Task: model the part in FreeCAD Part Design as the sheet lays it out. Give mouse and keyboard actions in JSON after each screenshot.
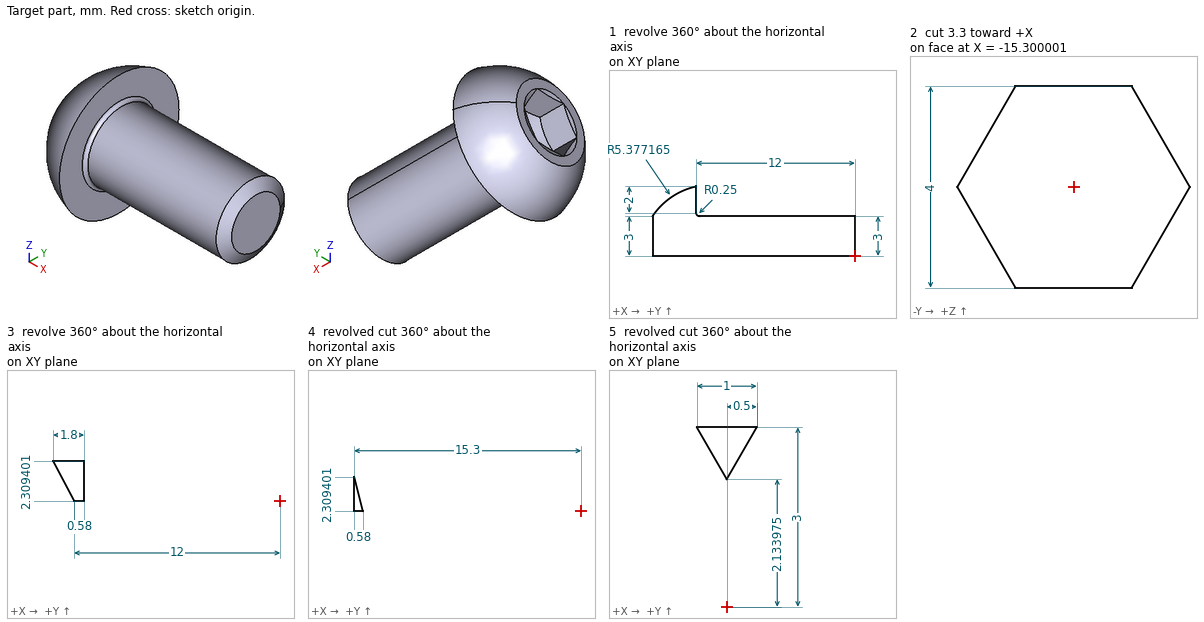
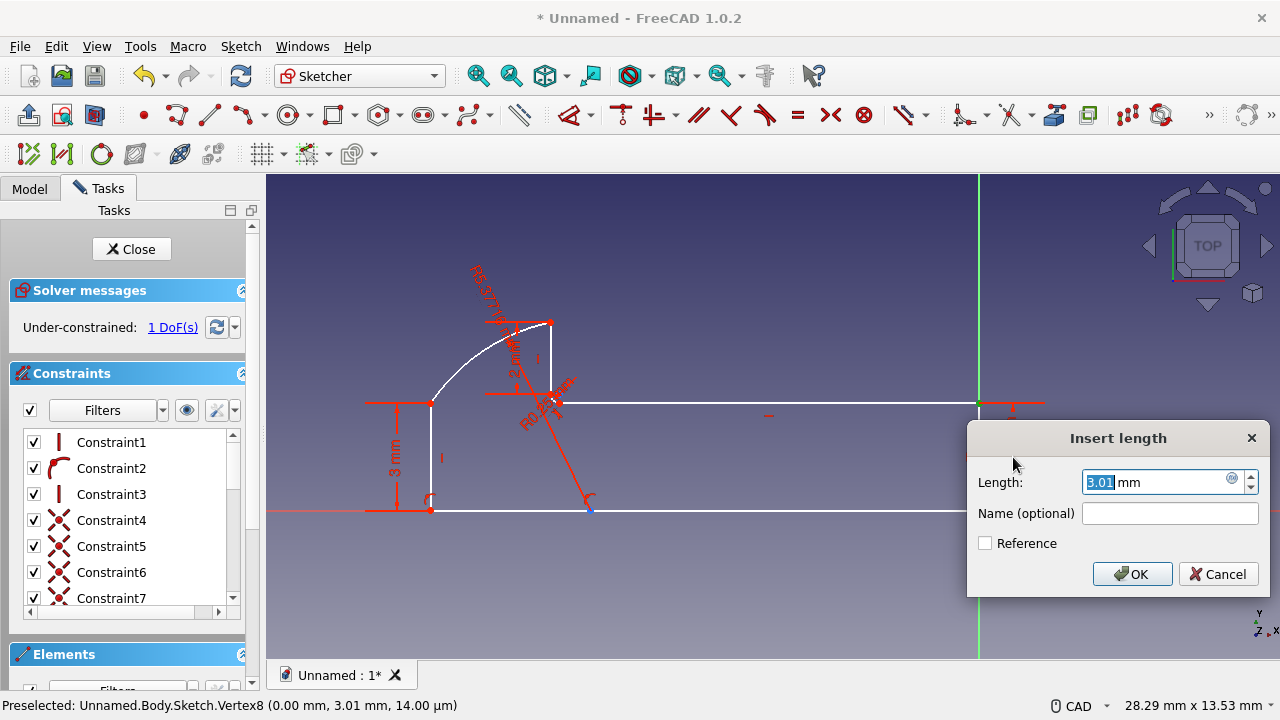
{"action": "type", "text": "3"}
{"action": "key", "text": "Return"}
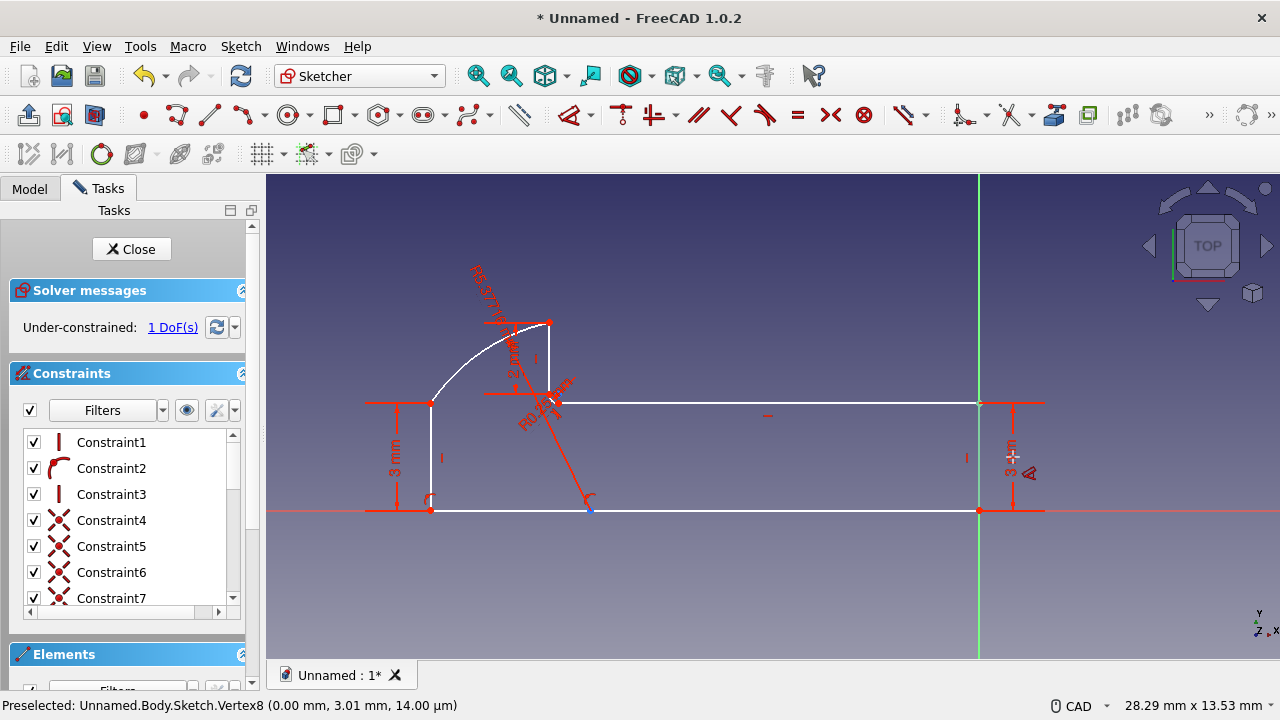
{"action": "scroll", "coordinate": [549, 394], "scroll_direction": "up", "scroll_amount": 2}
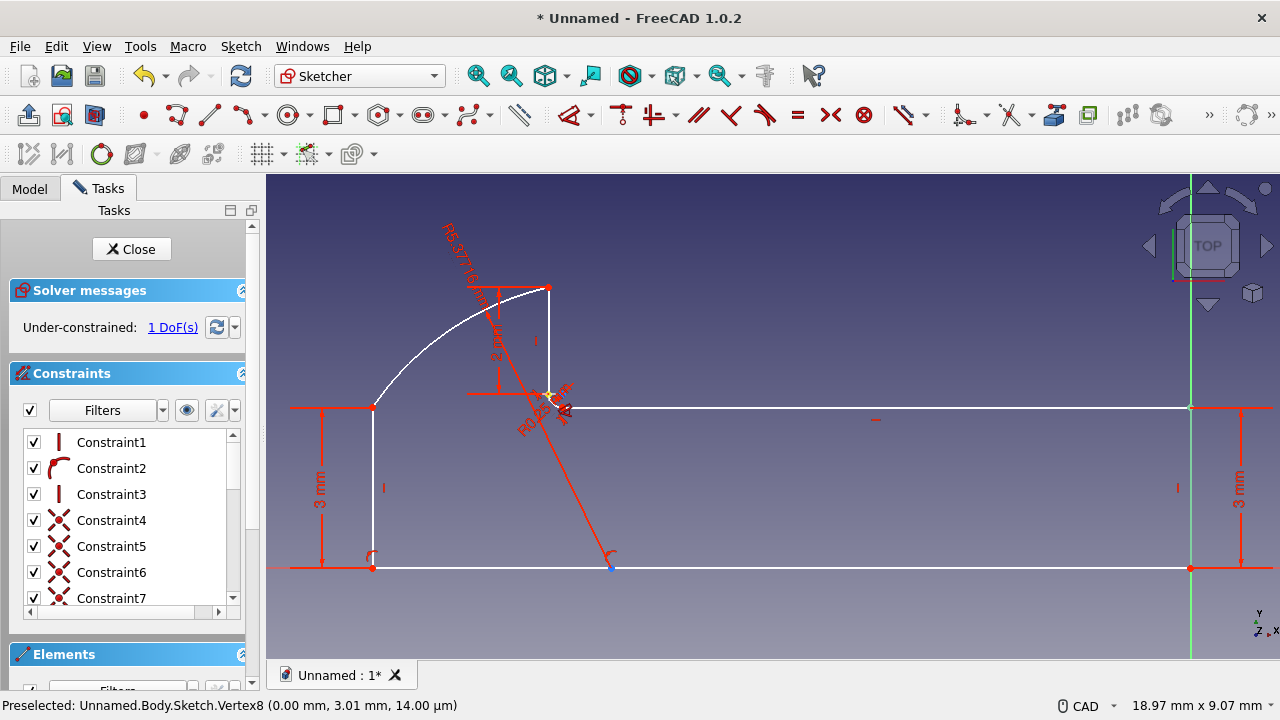
{"action": "left_click", "coordinate": [549, 394]}
{"action": "left_click", "coordinate": [832, 602]}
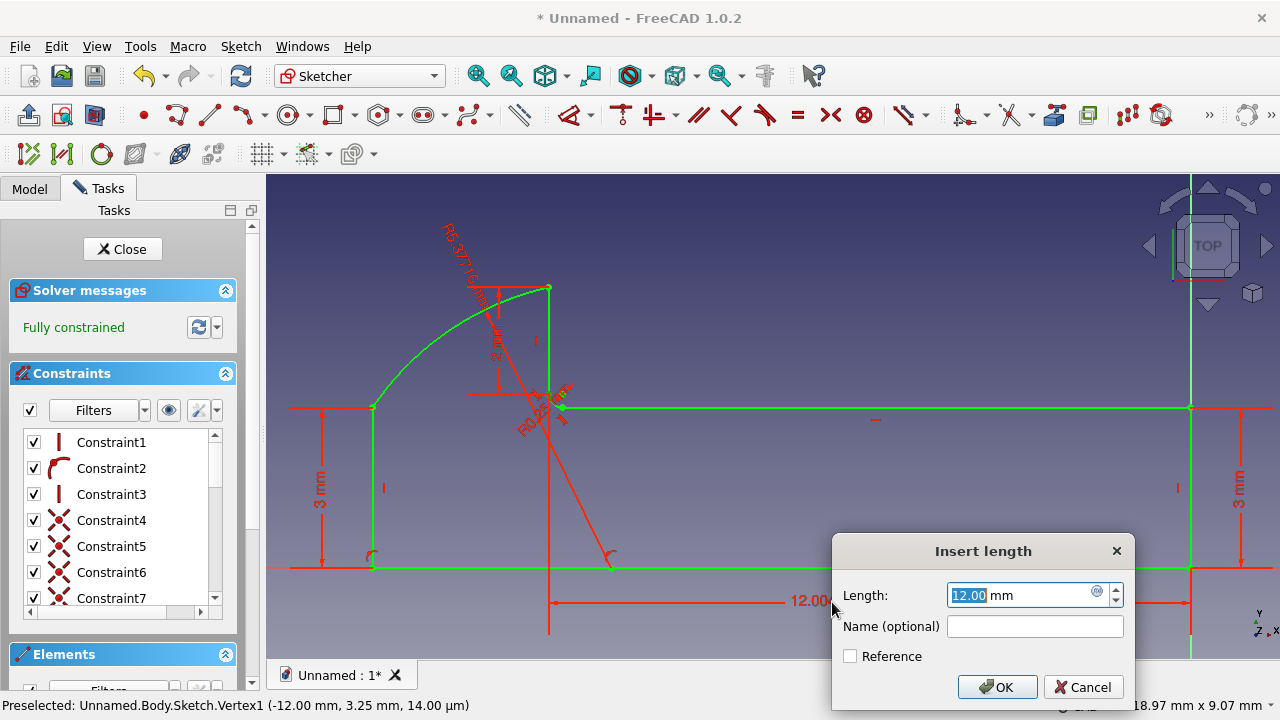
{"action": "type", "text": "12"}
{"action": "key", "text": "Return"}
{"action": "key", "text": "Escape"}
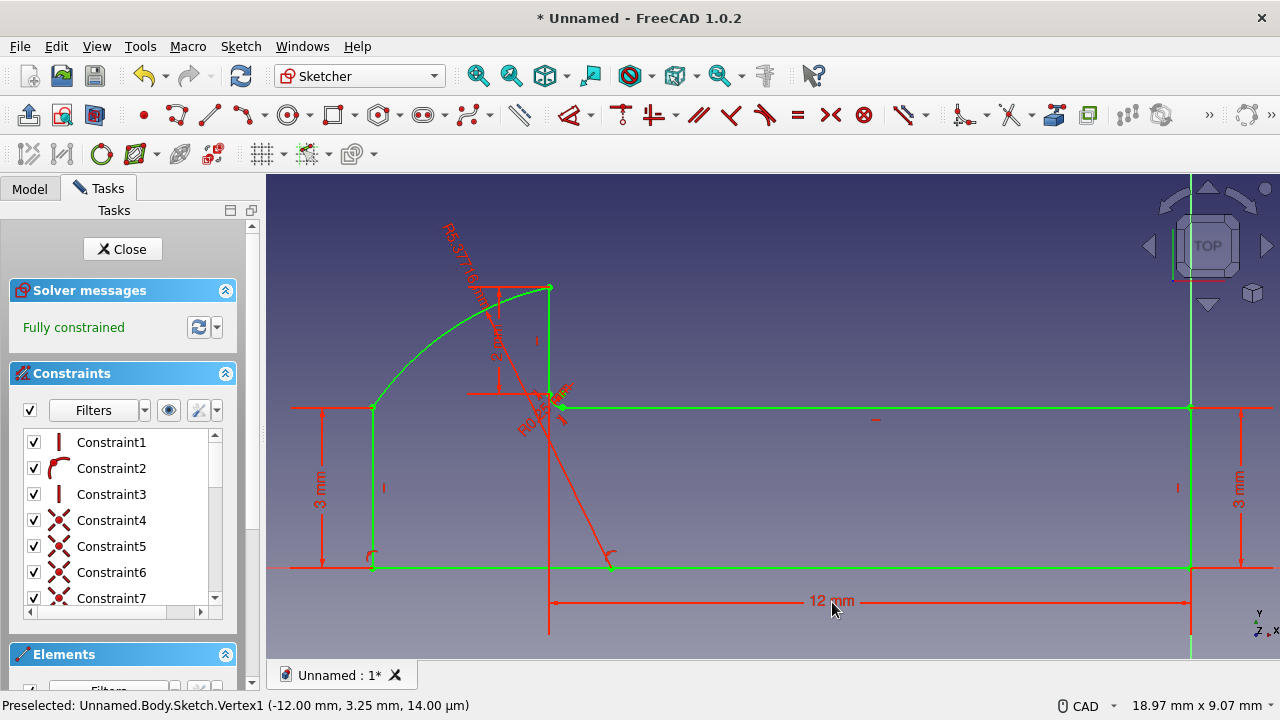
{"action": "left_click", "coordinate": [123, 249]}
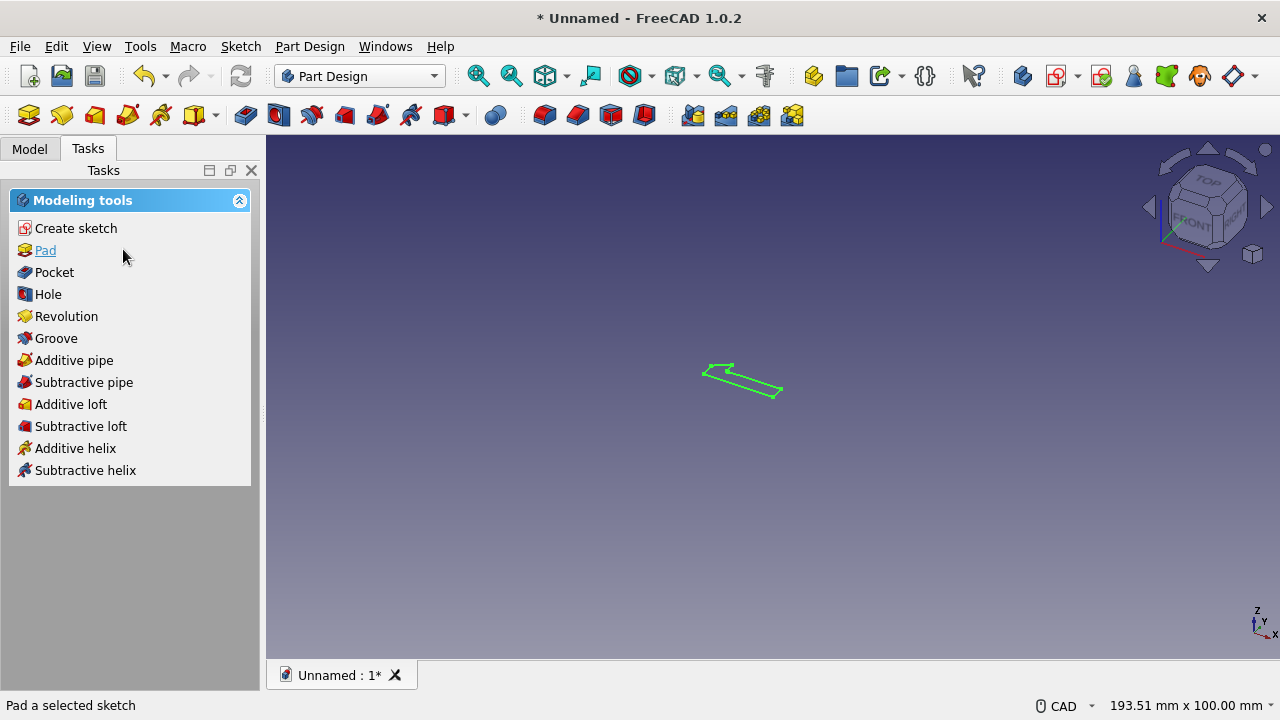
{"action": "left_click", "coordinate": [62, 116]}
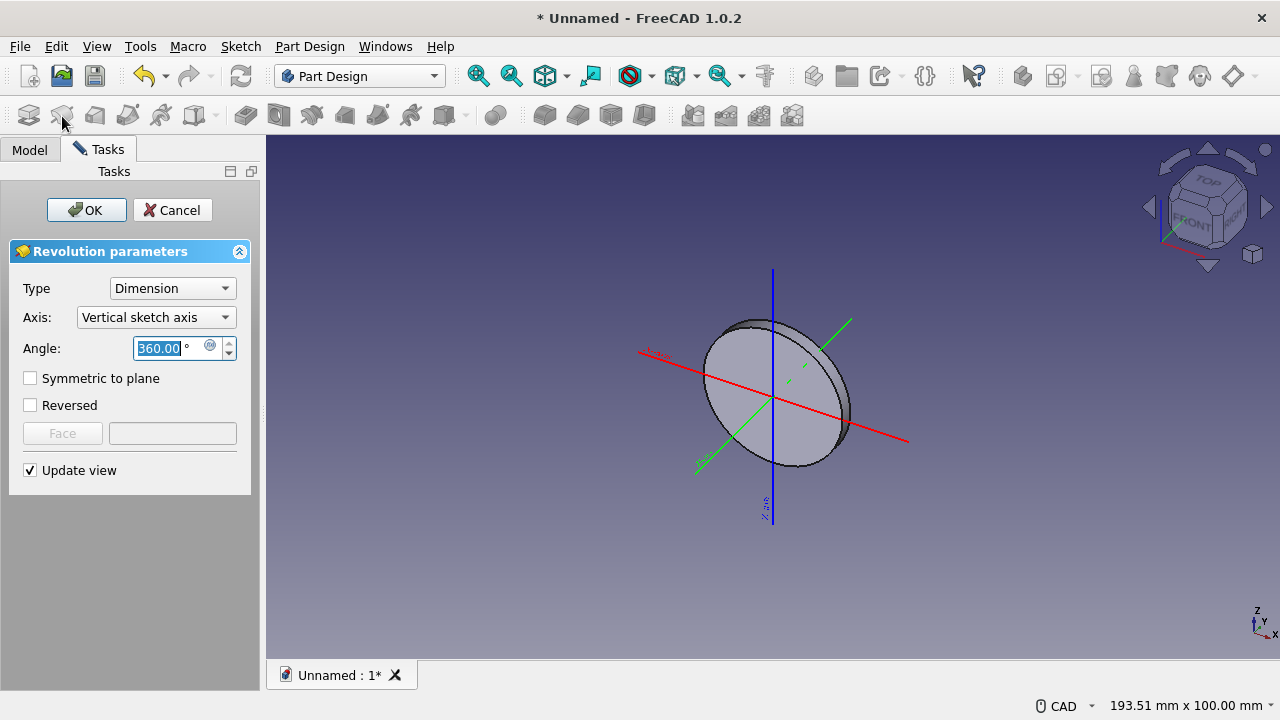
{"action": "left_click", "coordinate": [157, 318]}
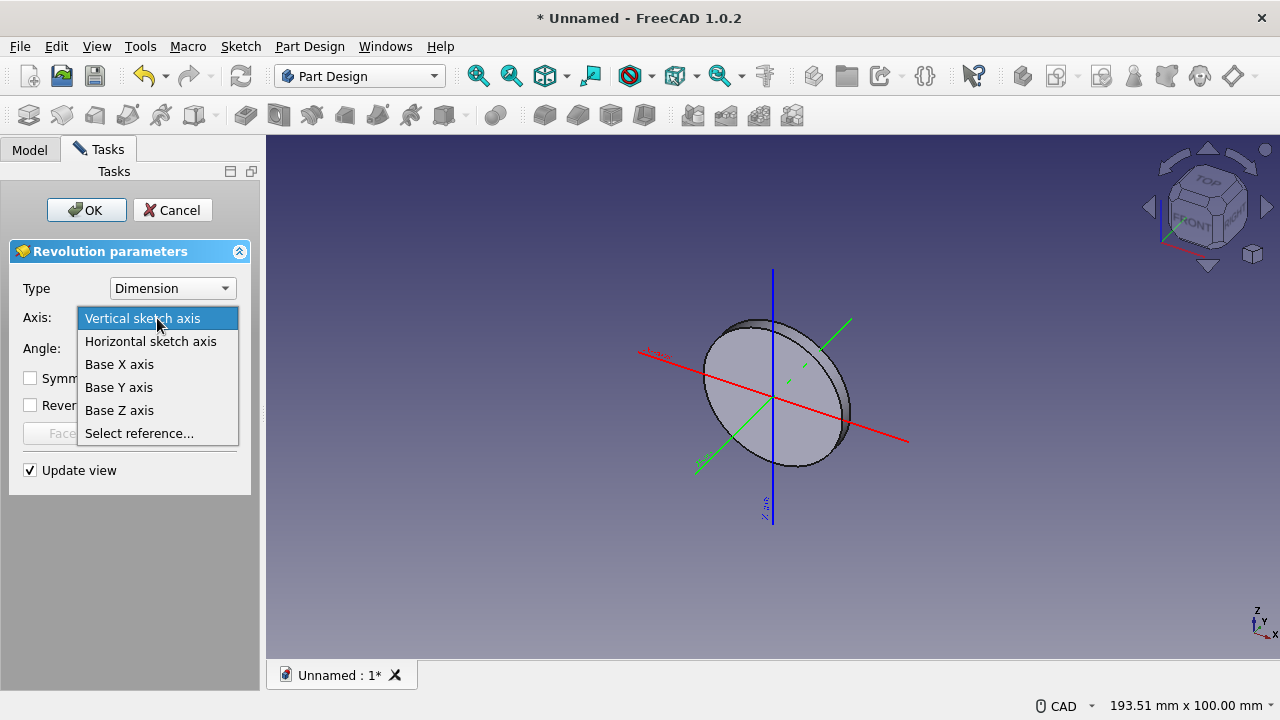
{"action": "left_click", "coordinate": [156, 342]}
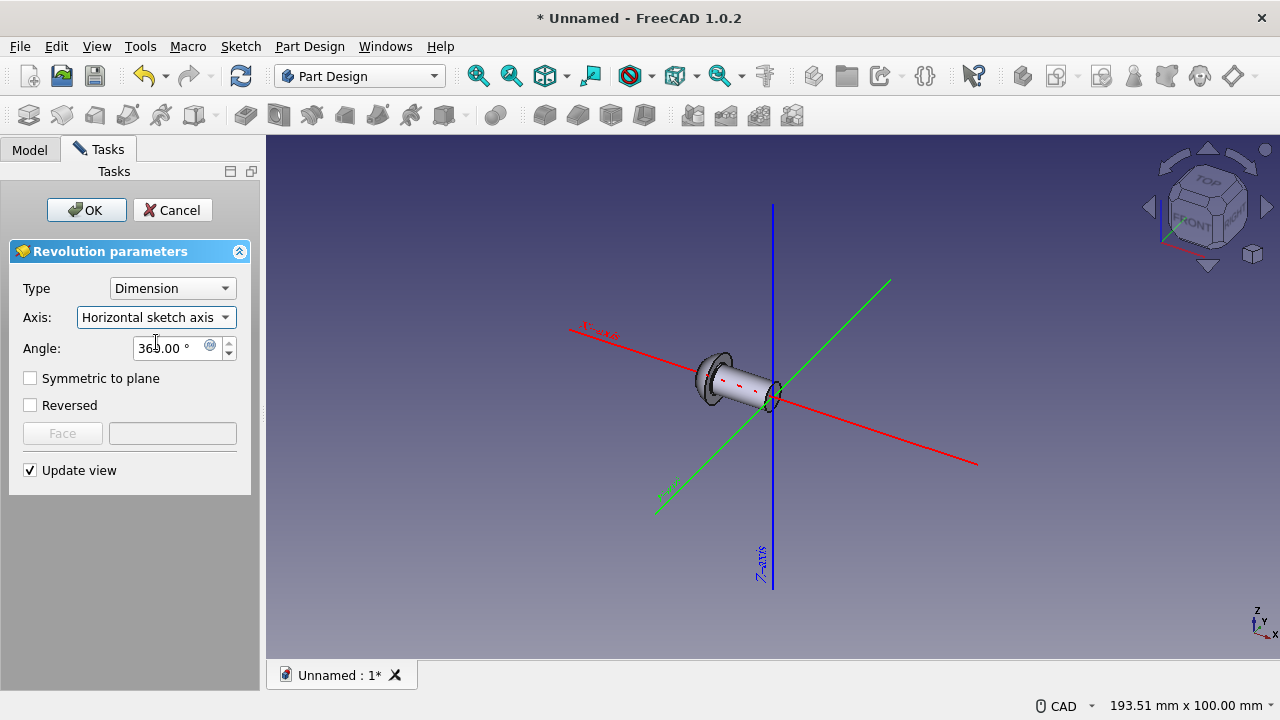
{"action": "left_click", "coordinate": [87, 210]}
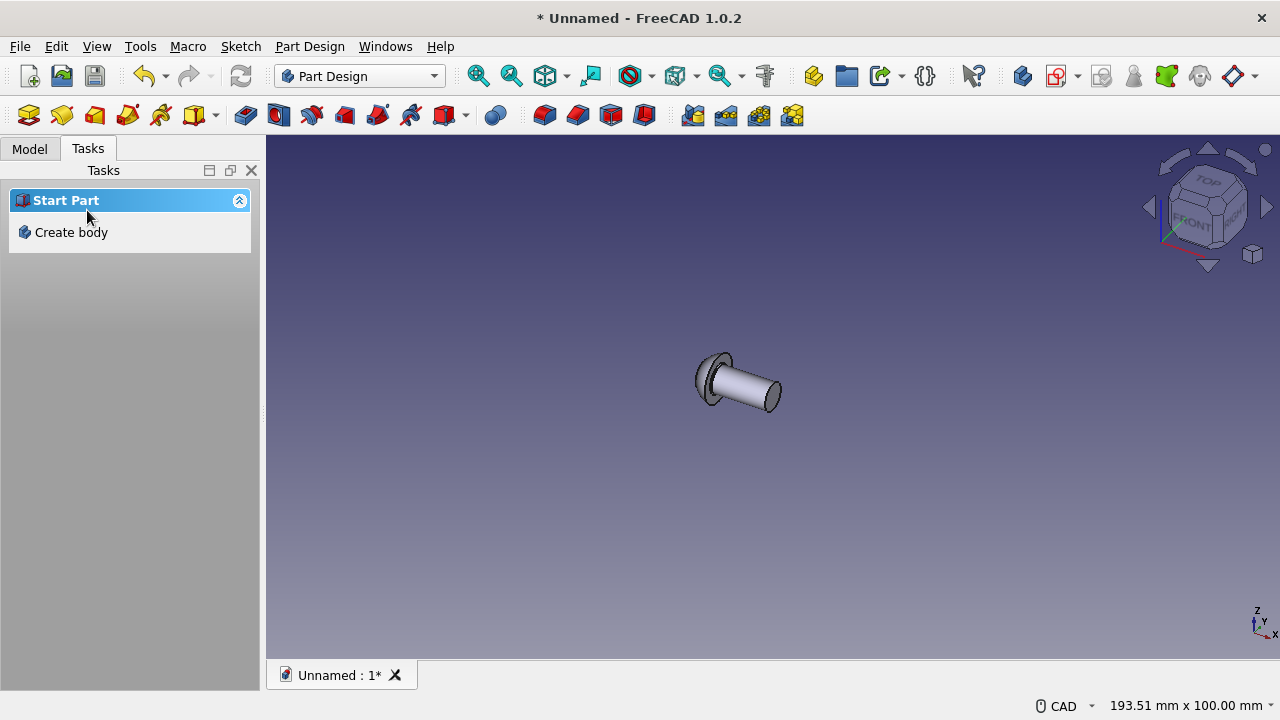
{"action": "left_click", "coordinate": [479, 76]}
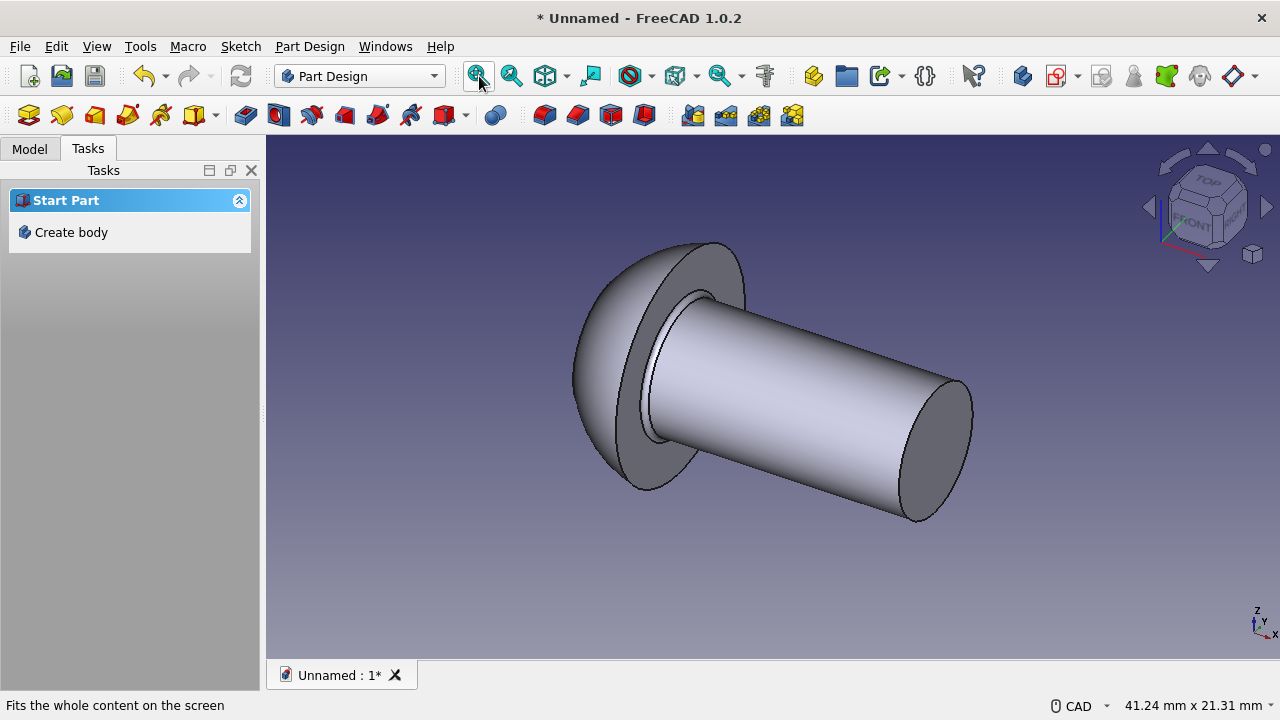
{"action": "key", "text": "6"}